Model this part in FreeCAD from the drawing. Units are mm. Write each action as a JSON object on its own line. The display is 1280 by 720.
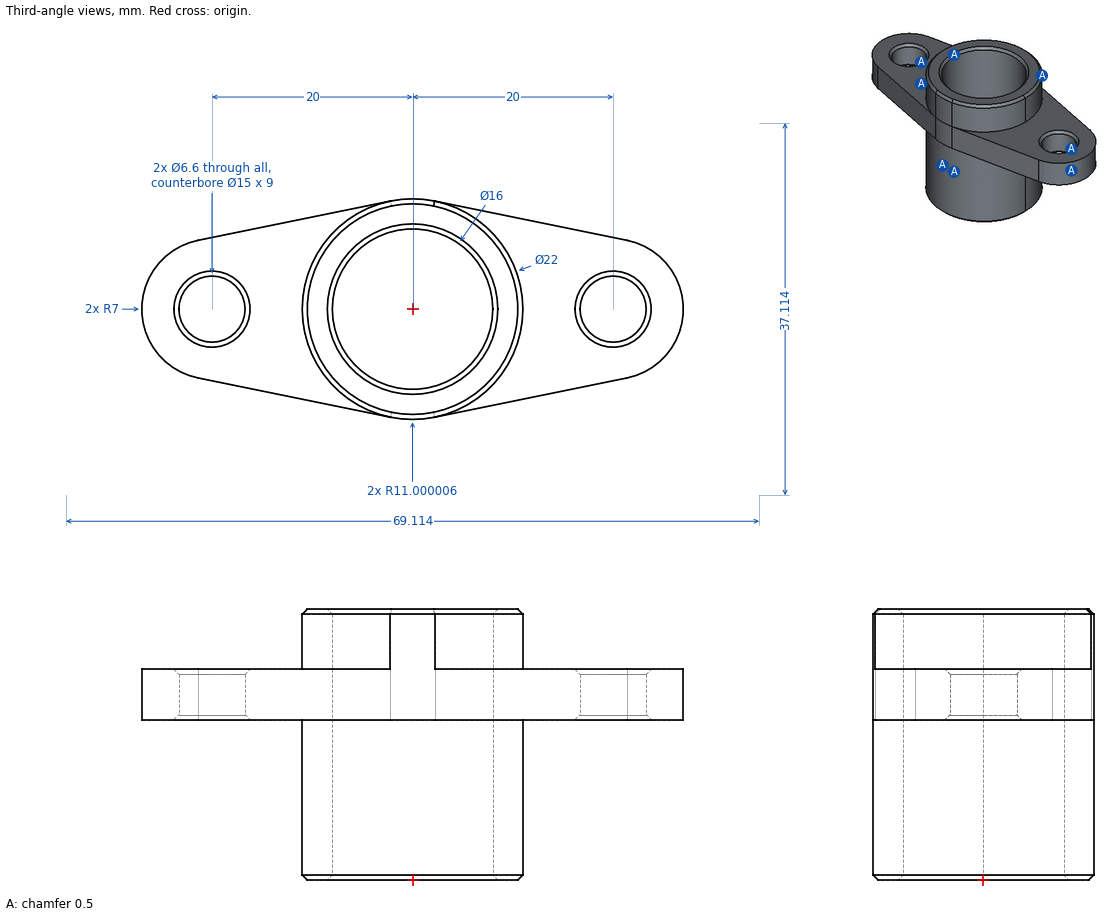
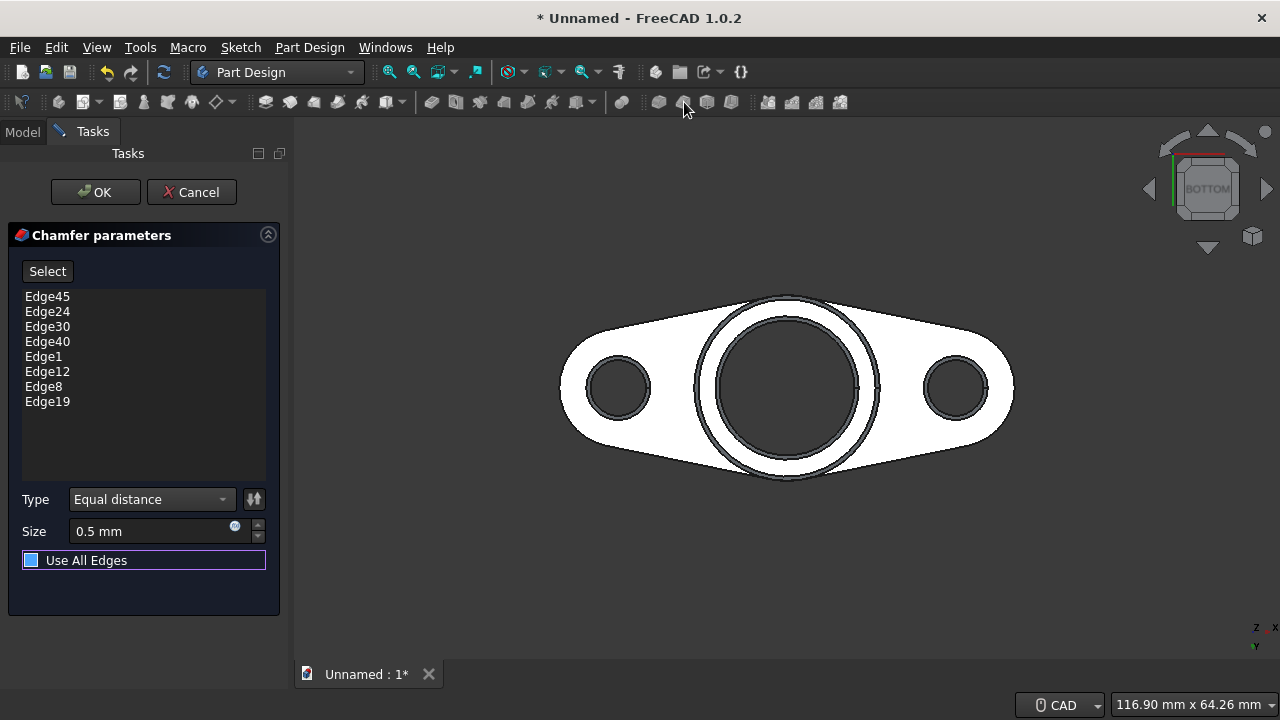
{"action": "left_click", "coordinate": [96, 192]}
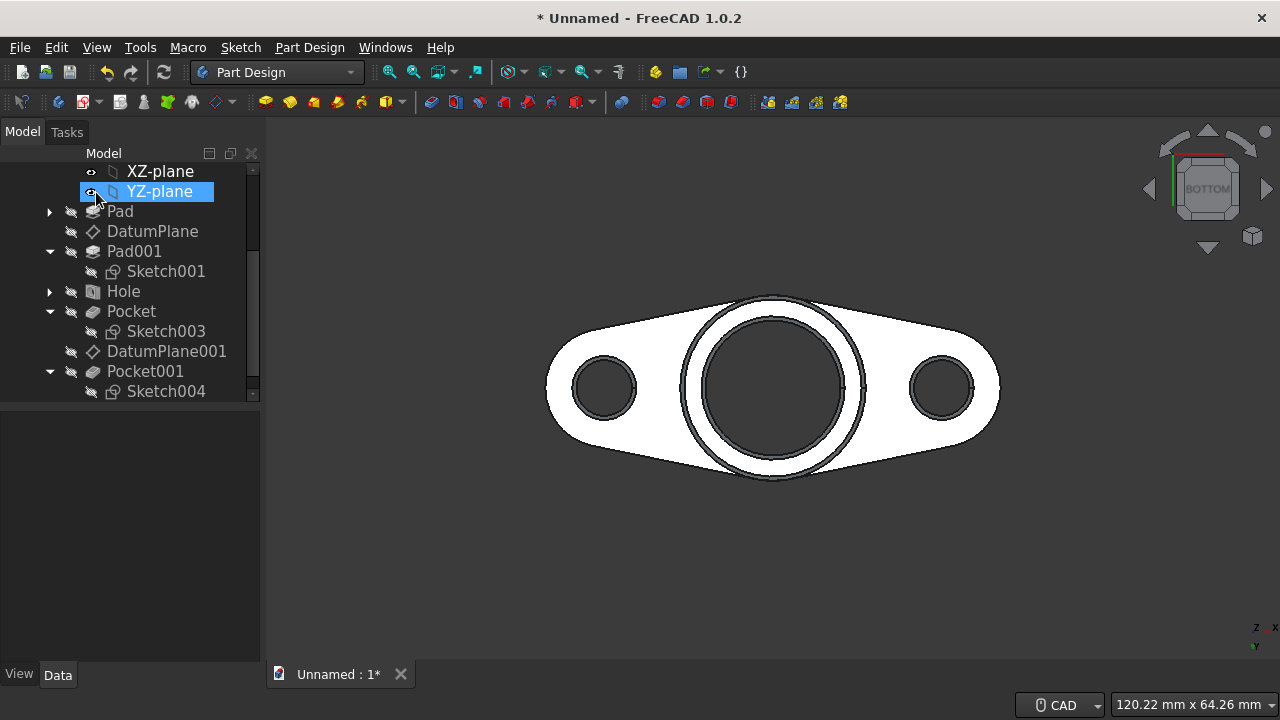
{"action": "key", "text": "0"}